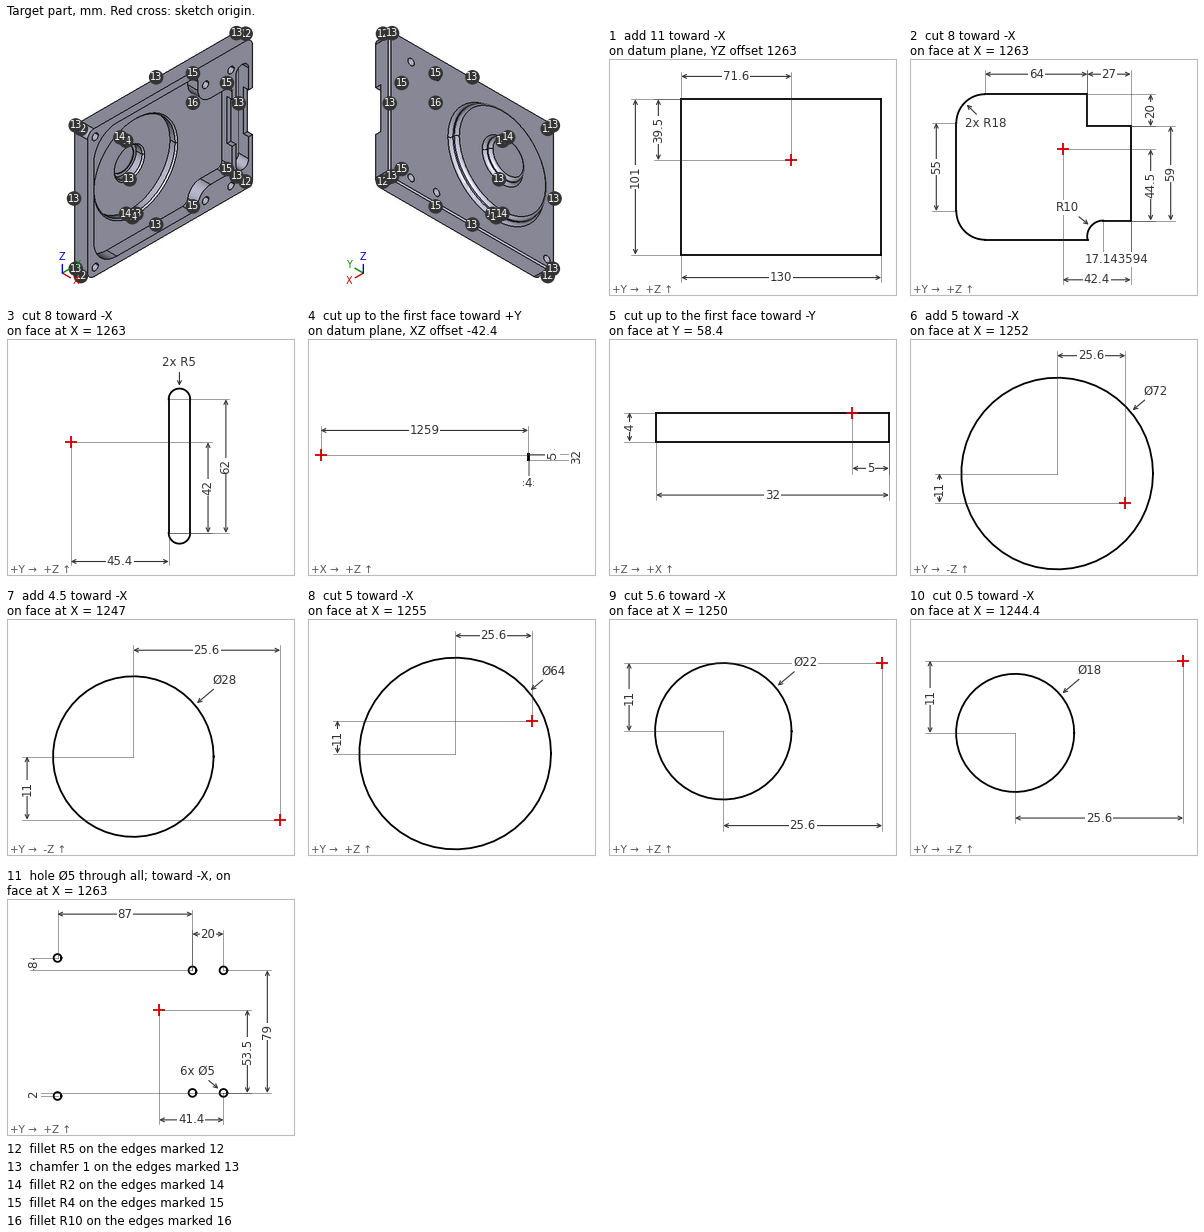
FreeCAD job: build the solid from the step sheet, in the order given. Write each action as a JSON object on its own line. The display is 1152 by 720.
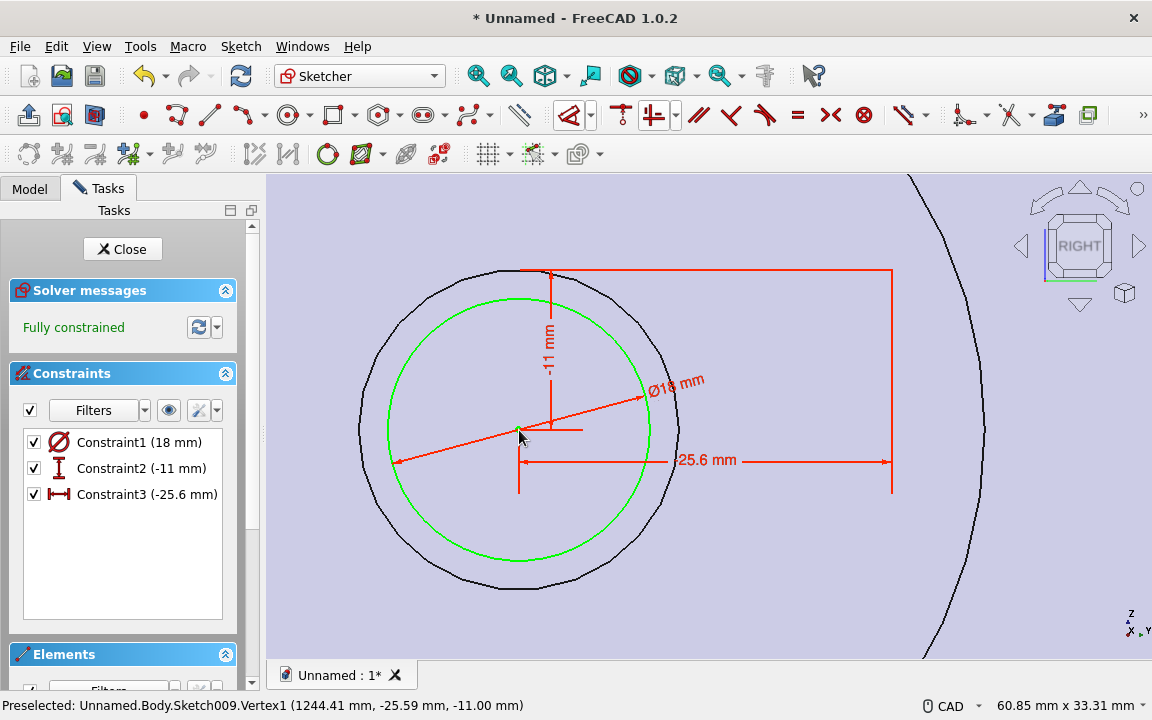
{"action": "left_click", "coordinate": [123, 249]}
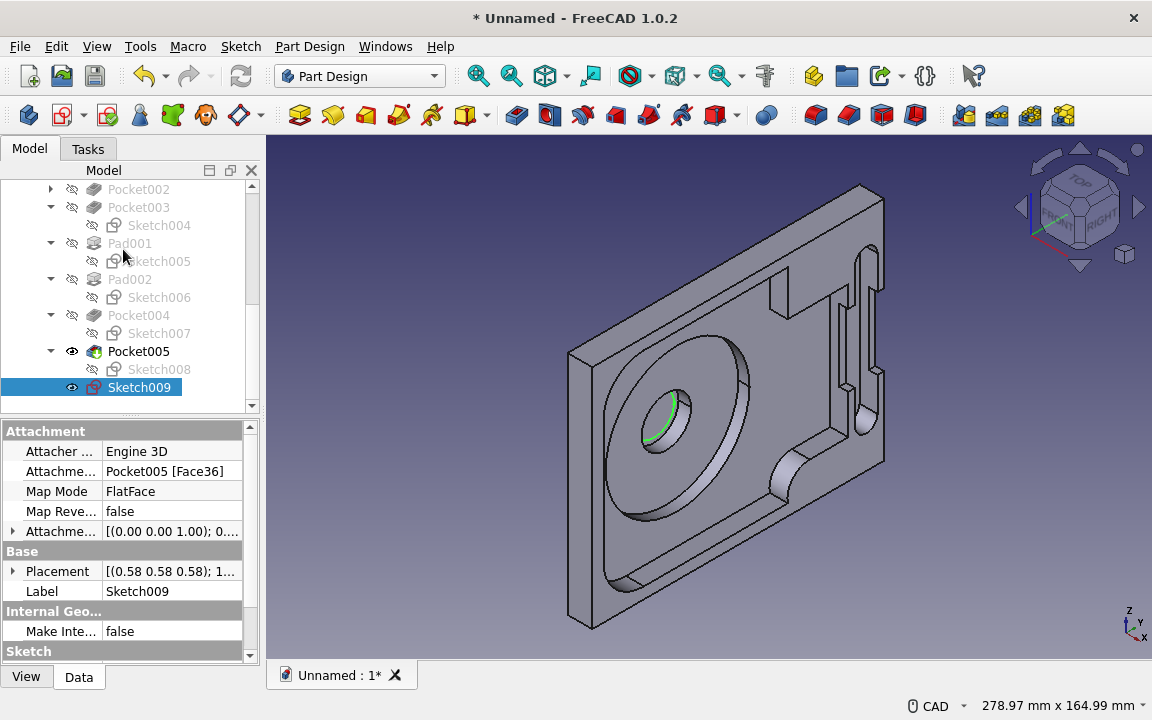
{"action": "left_click", "coordinate": [517, 116]}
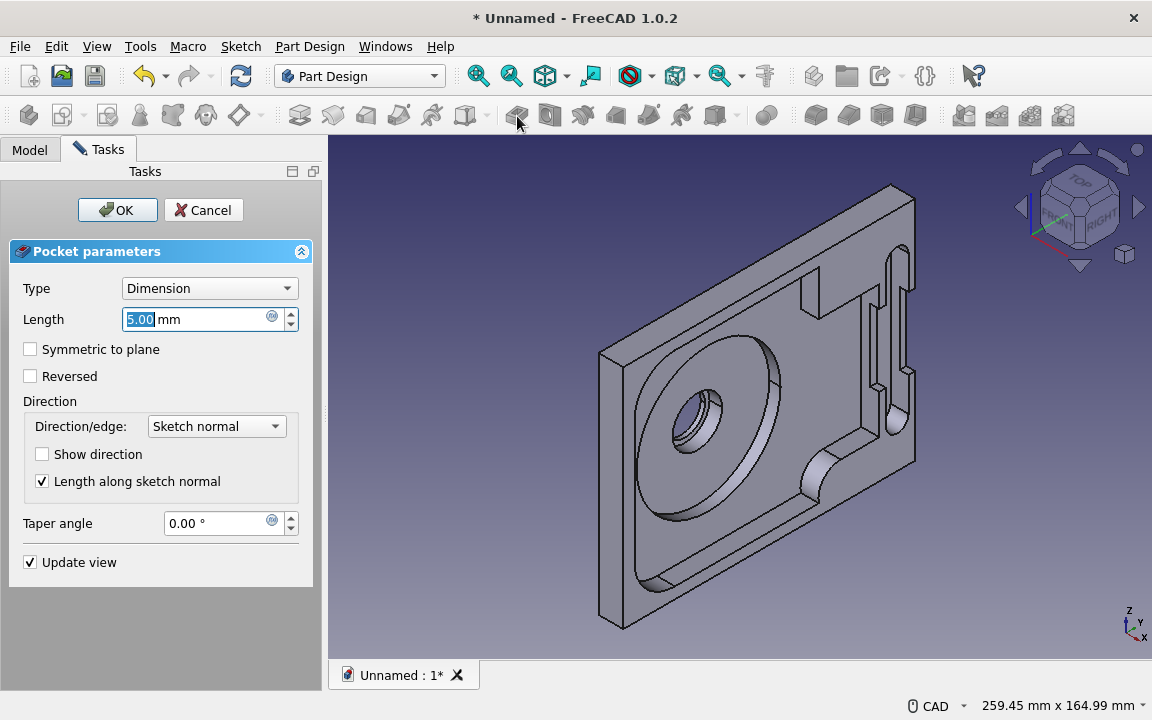
{"action": "type", "text": "0.5"}
{"action": "key", "text": "Tab"}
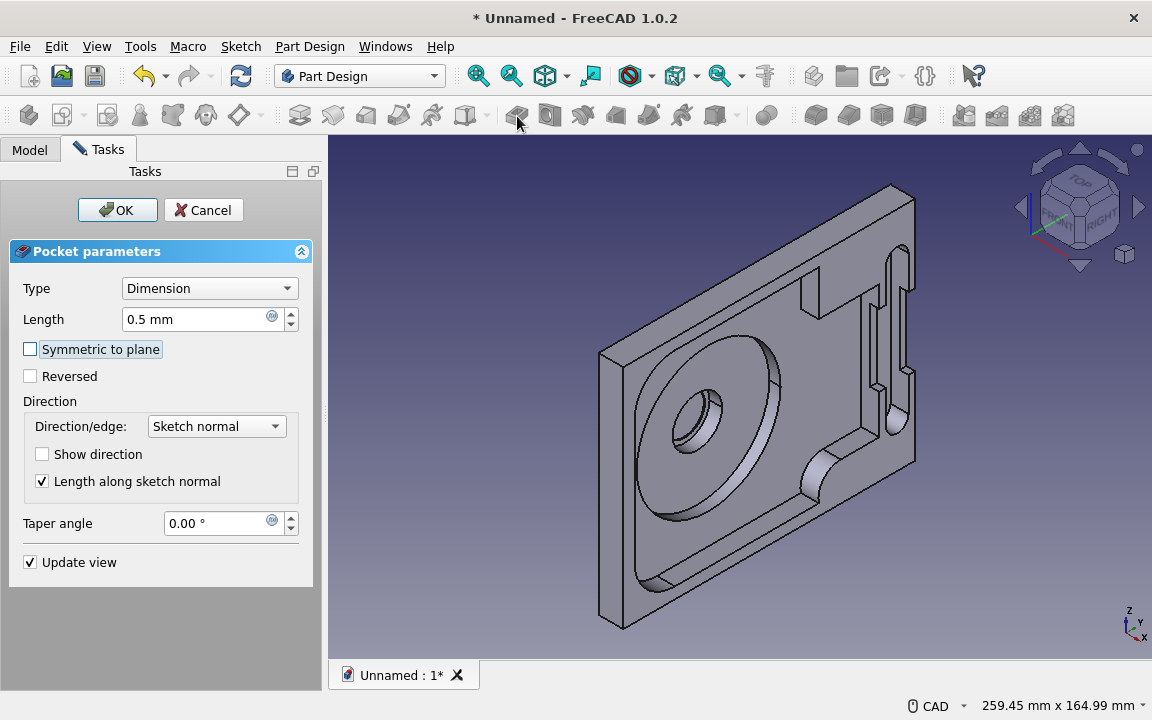
{"action": "left_click", "coordinate": [118, 210]}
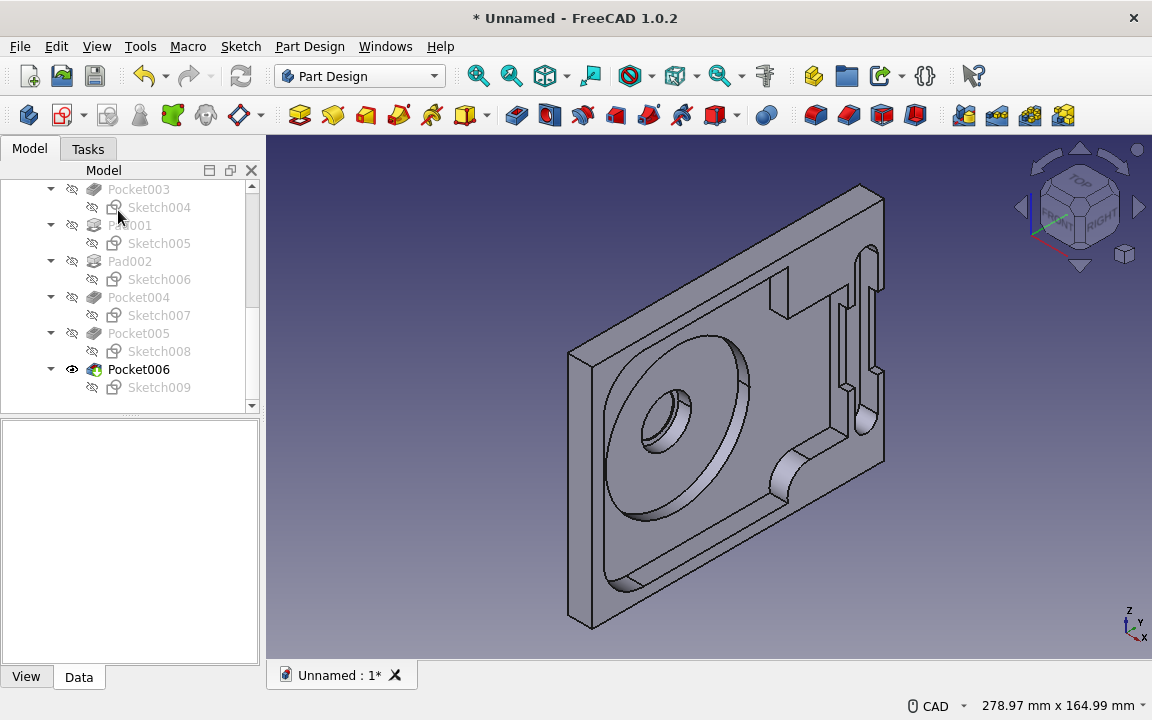
{"action": "left_click", "coordinate": [863, 228]}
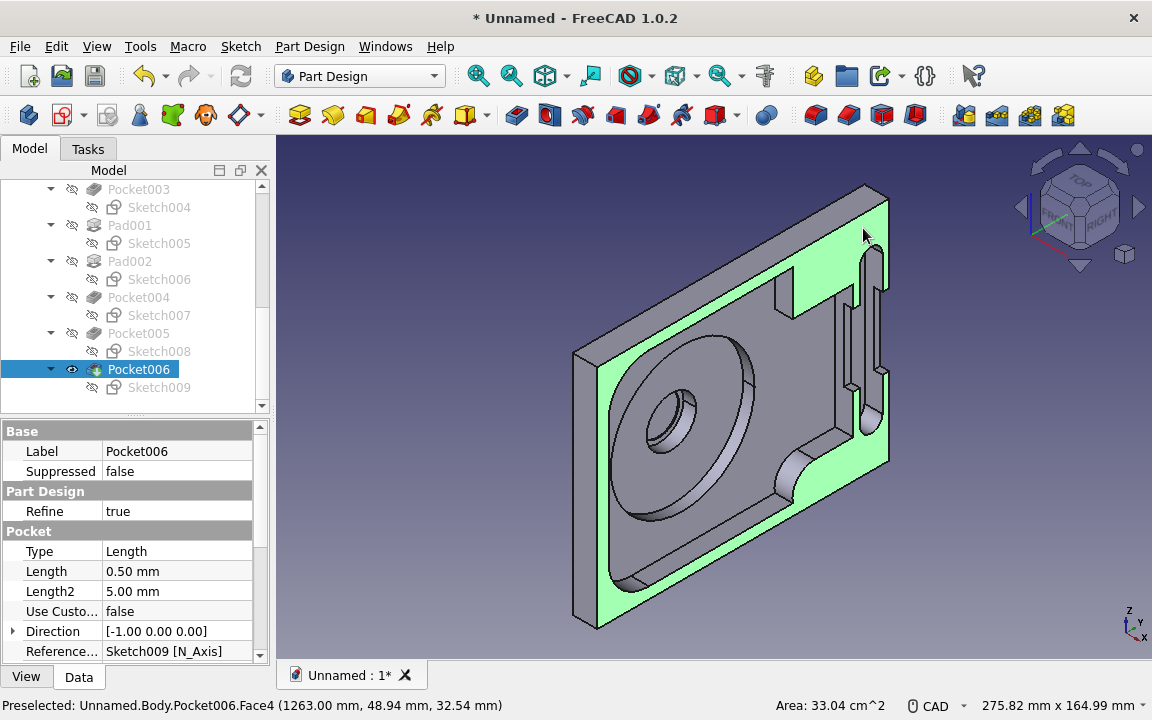
{"action": "left_click", "coordinate": [62, 116]}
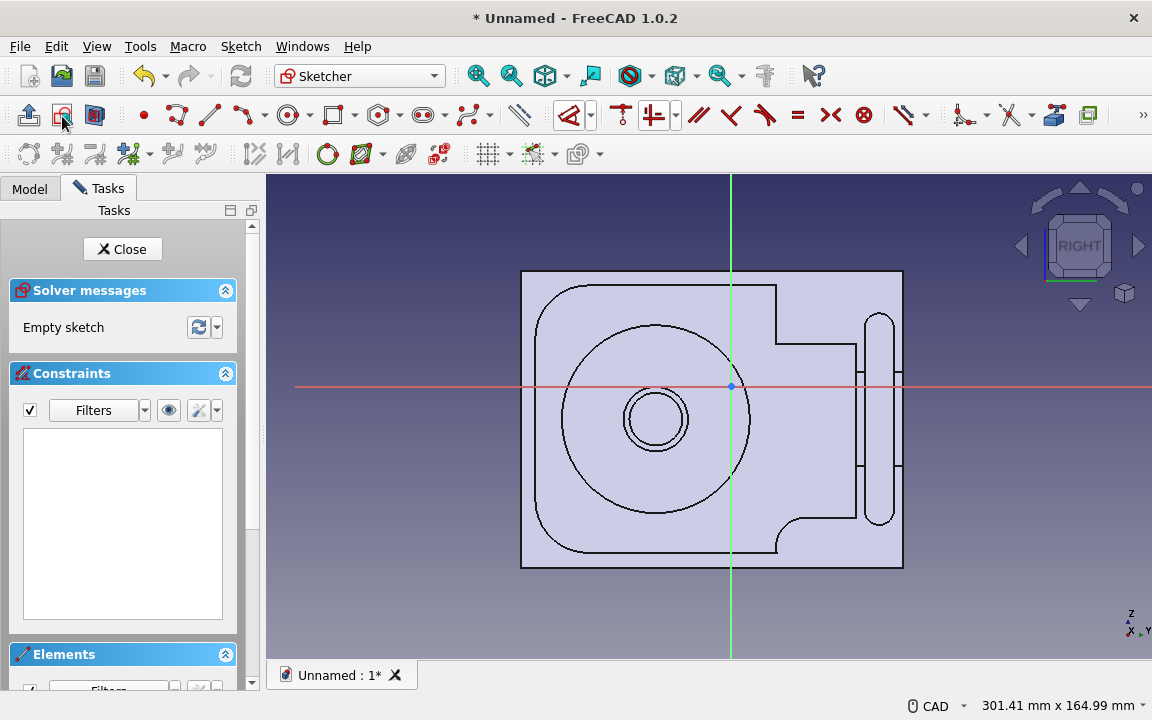
{"action": "left_click", "coordinate": [288, 116]}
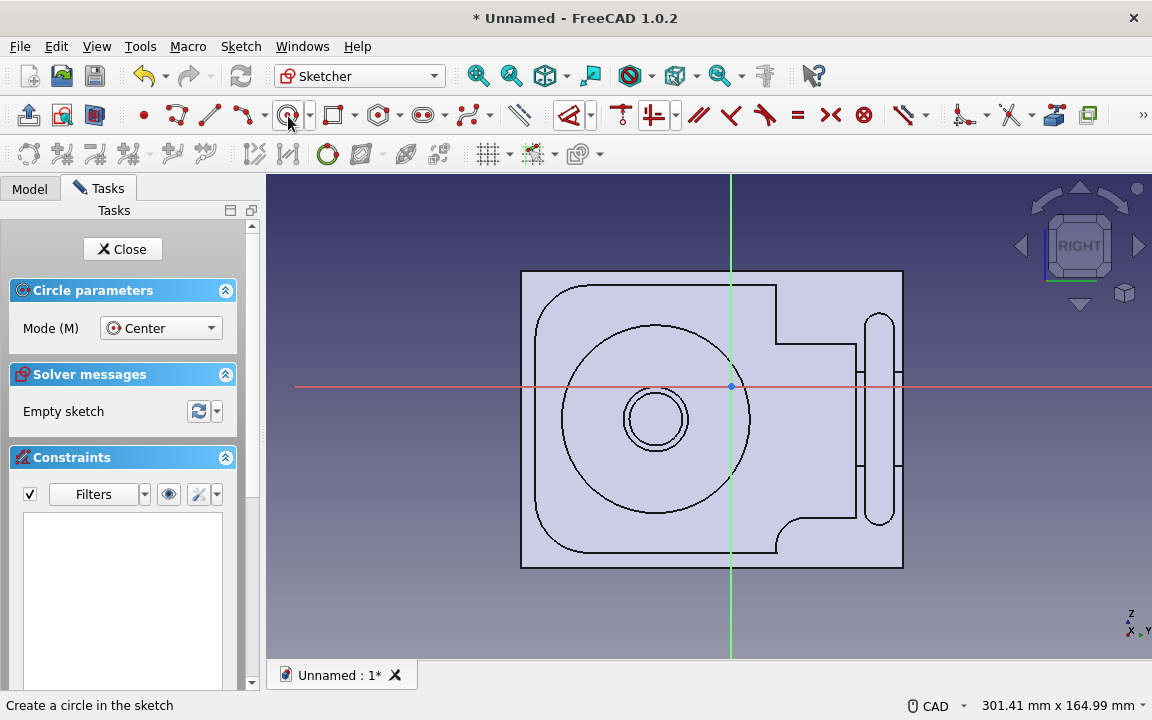
{"action": "scroll", "coordinate": [853, 544], "scroll_direction": "up", "scroll_amount": 6}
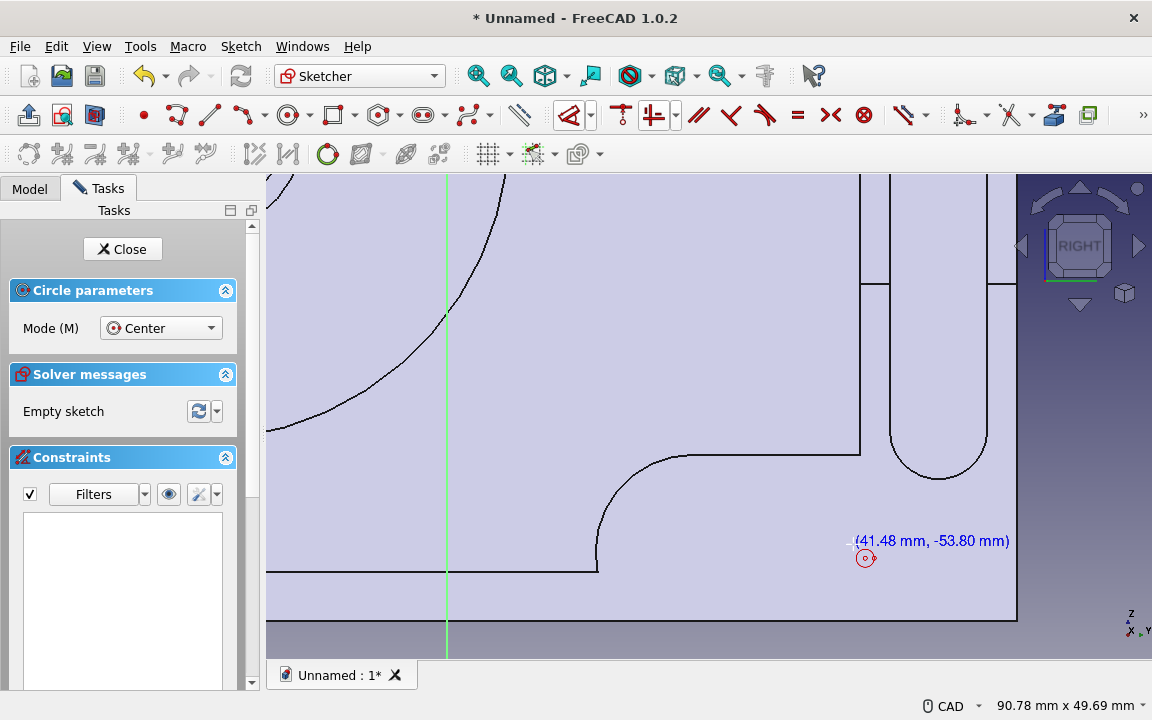
{"action": "left_click", "coordinate": [851, 543]}
{"action": "left_click", "coordinate": [868, 525]}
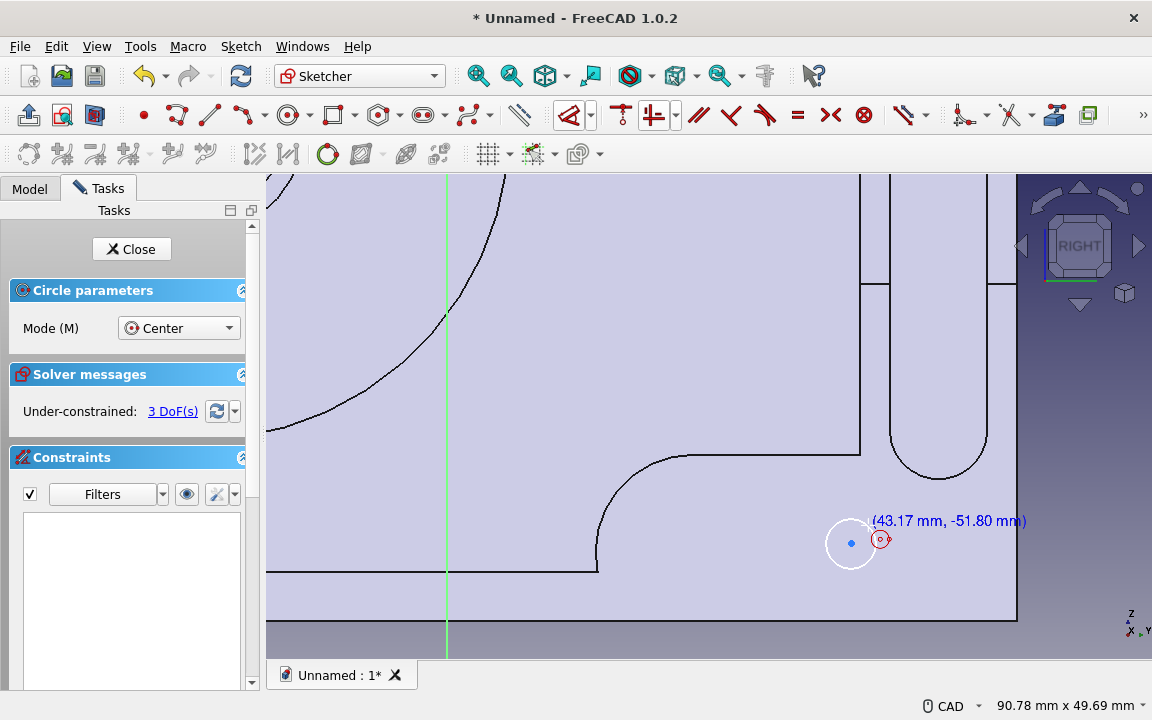
{"action": "scroll", "coordinate": [775, 541], "scroll_direction": "down", "scroll_amount": 6}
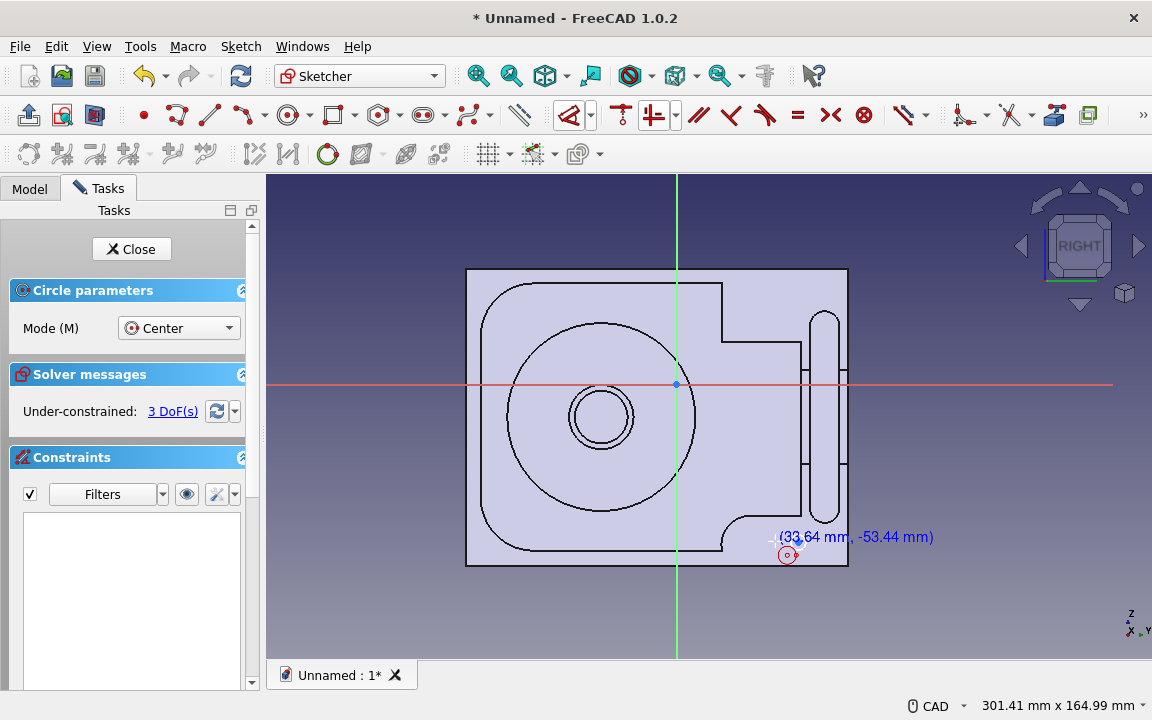
{"action": "scroll", "coordinate": [798, 310], "scroll_direction": "up", "scroll_amount": 6}